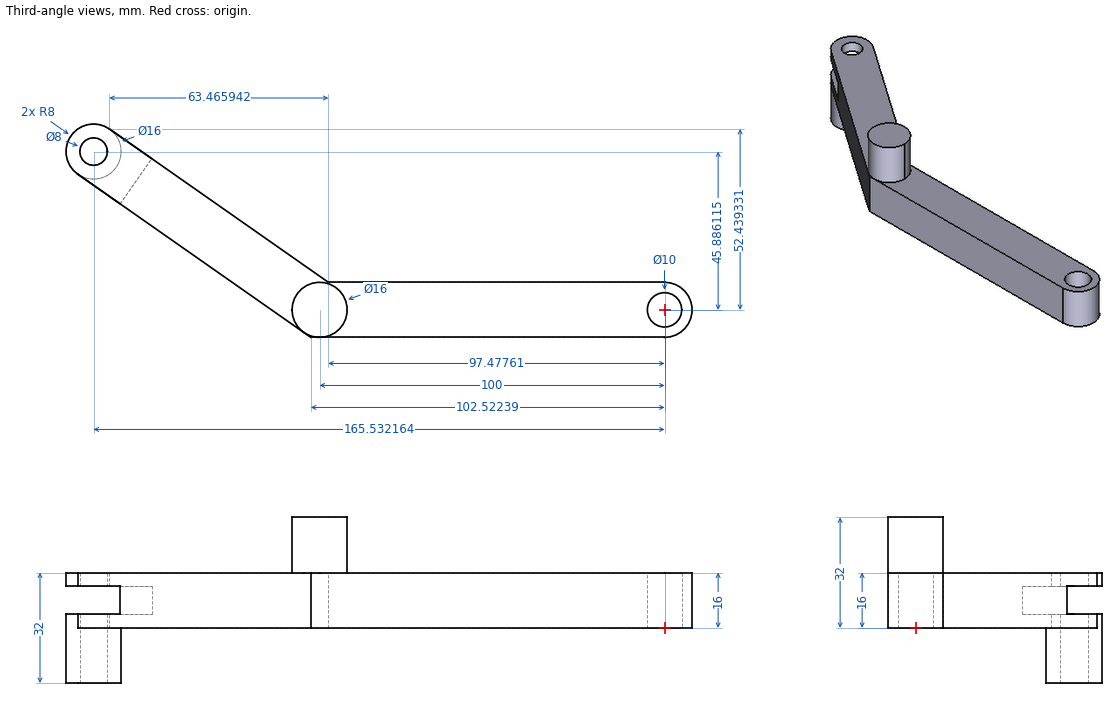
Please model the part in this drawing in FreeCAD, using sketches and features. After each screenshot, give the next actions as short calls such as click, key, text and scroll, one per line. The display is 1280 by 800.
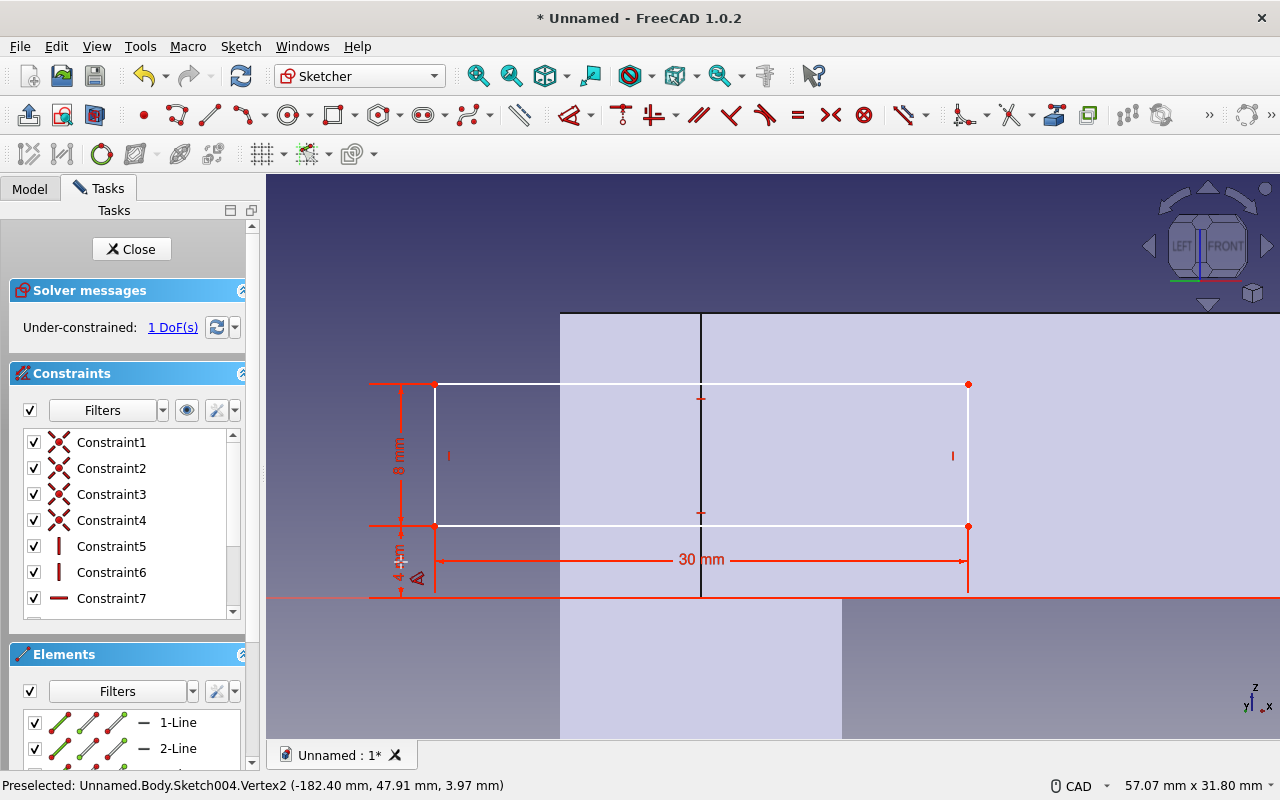
click(435, 384)
click(775, 632)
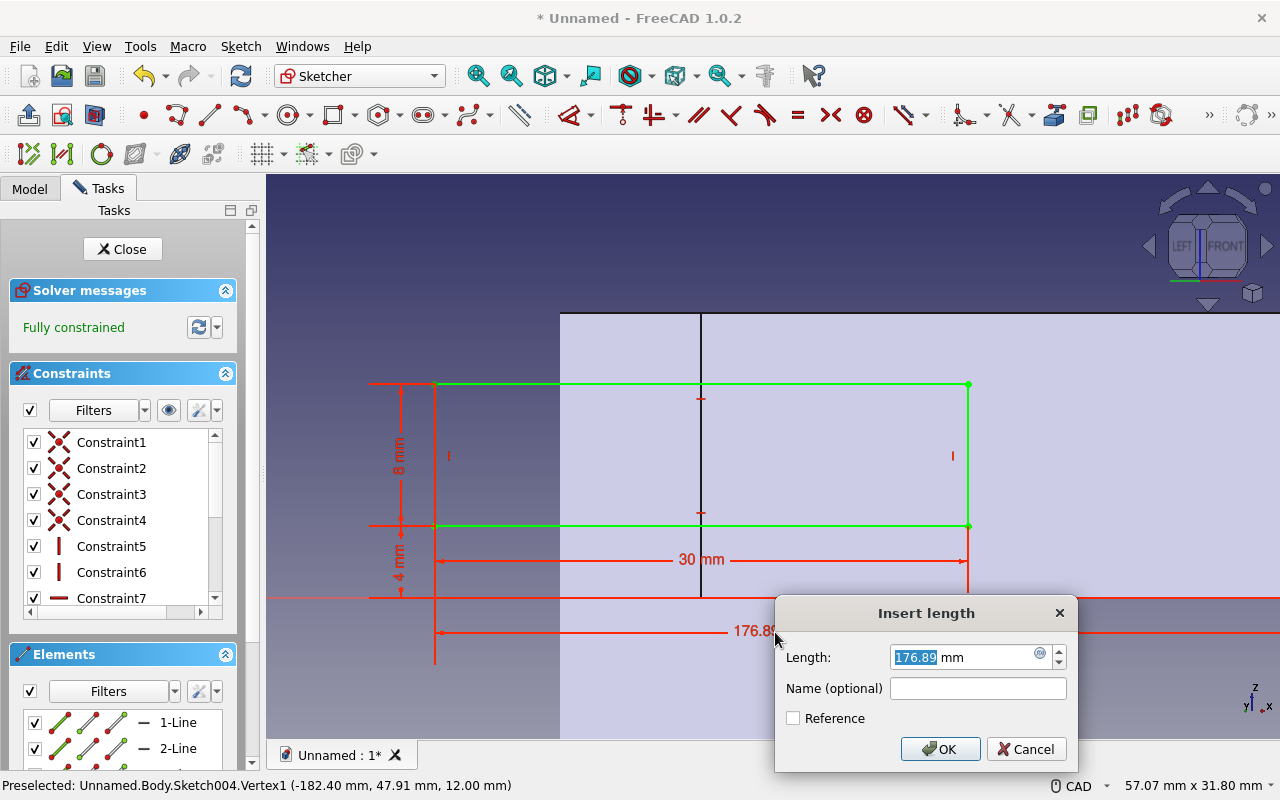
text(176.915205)
key(Return)
key(Escape)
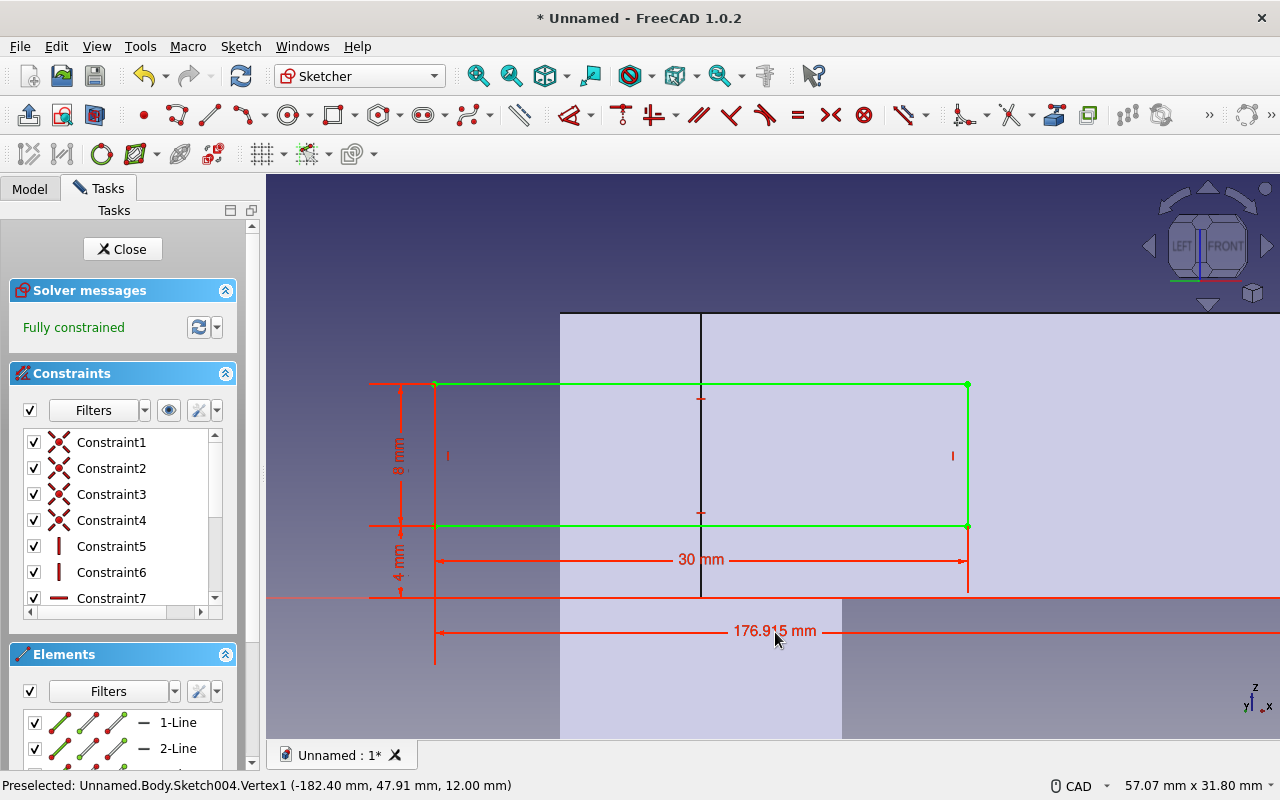
click(123, 249)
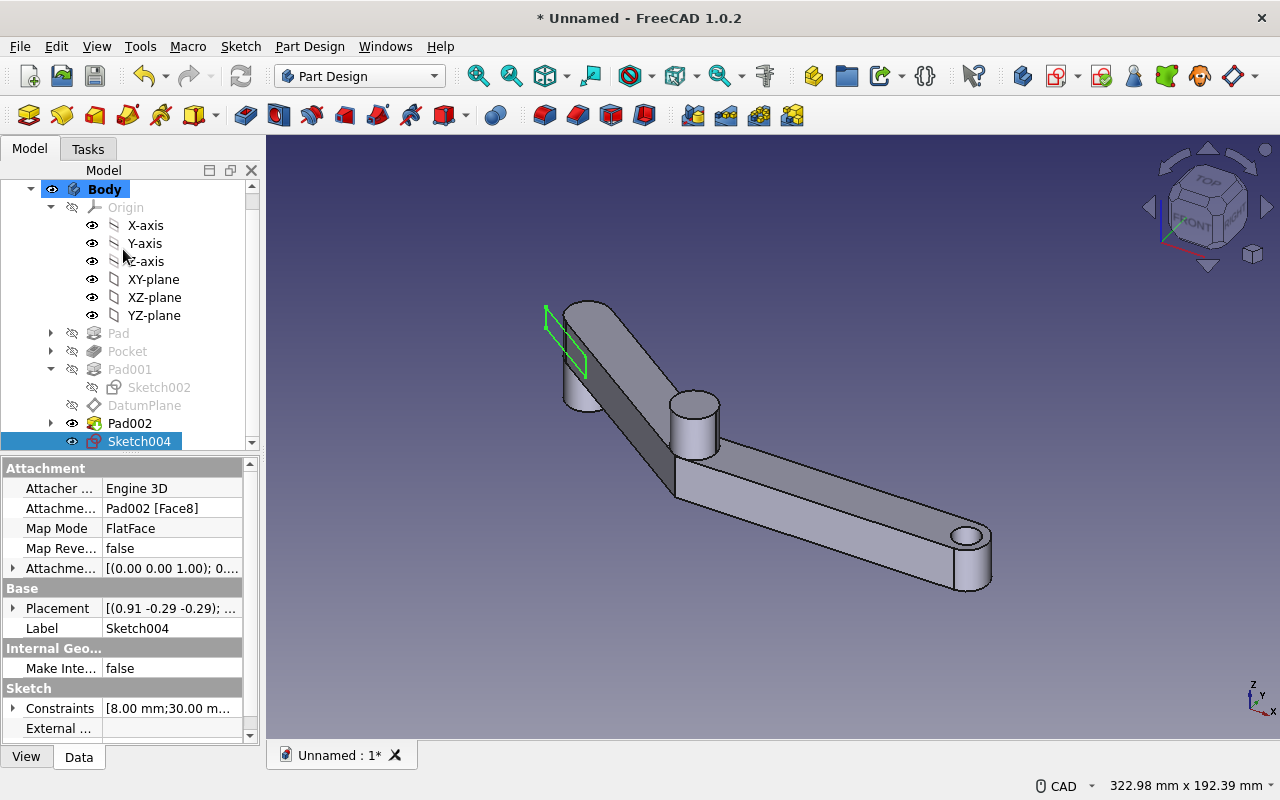
click(246, 116)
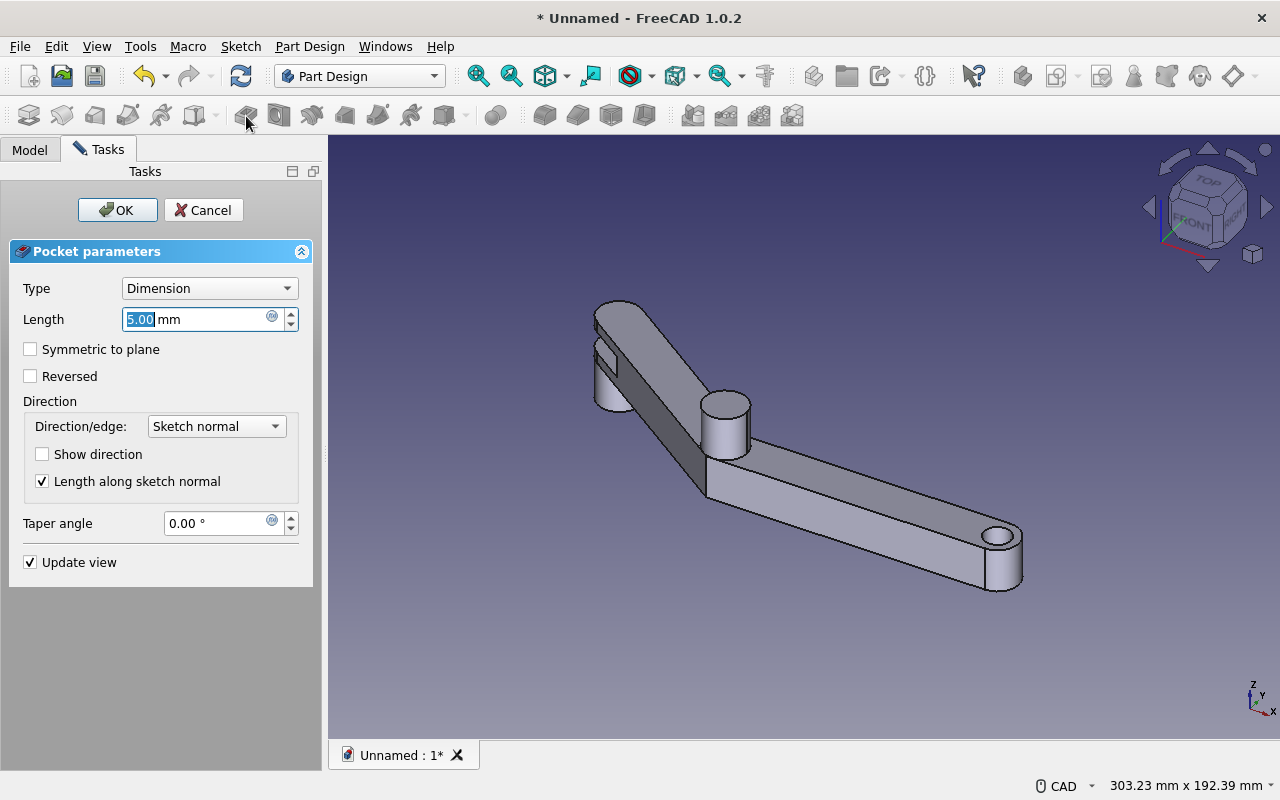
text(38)
key(Tab)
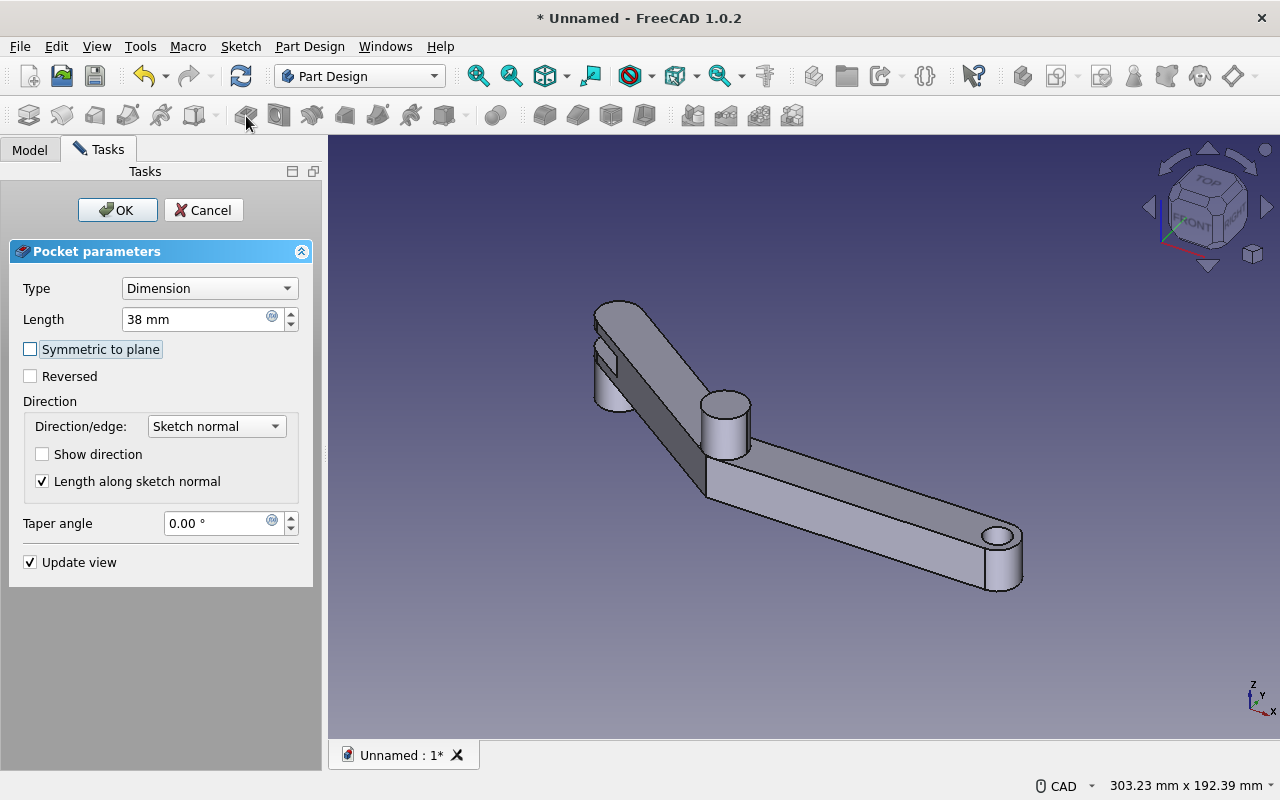
click(118, 210)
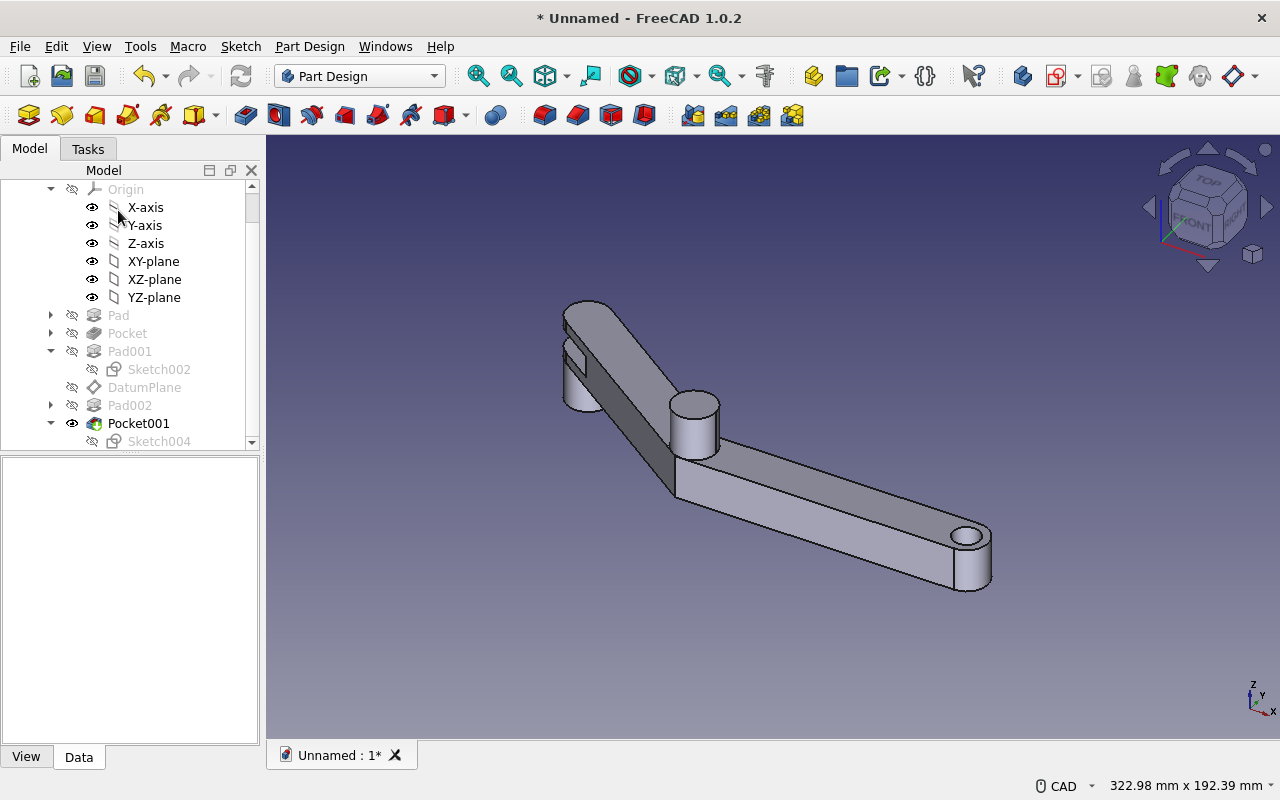
click(636, 378)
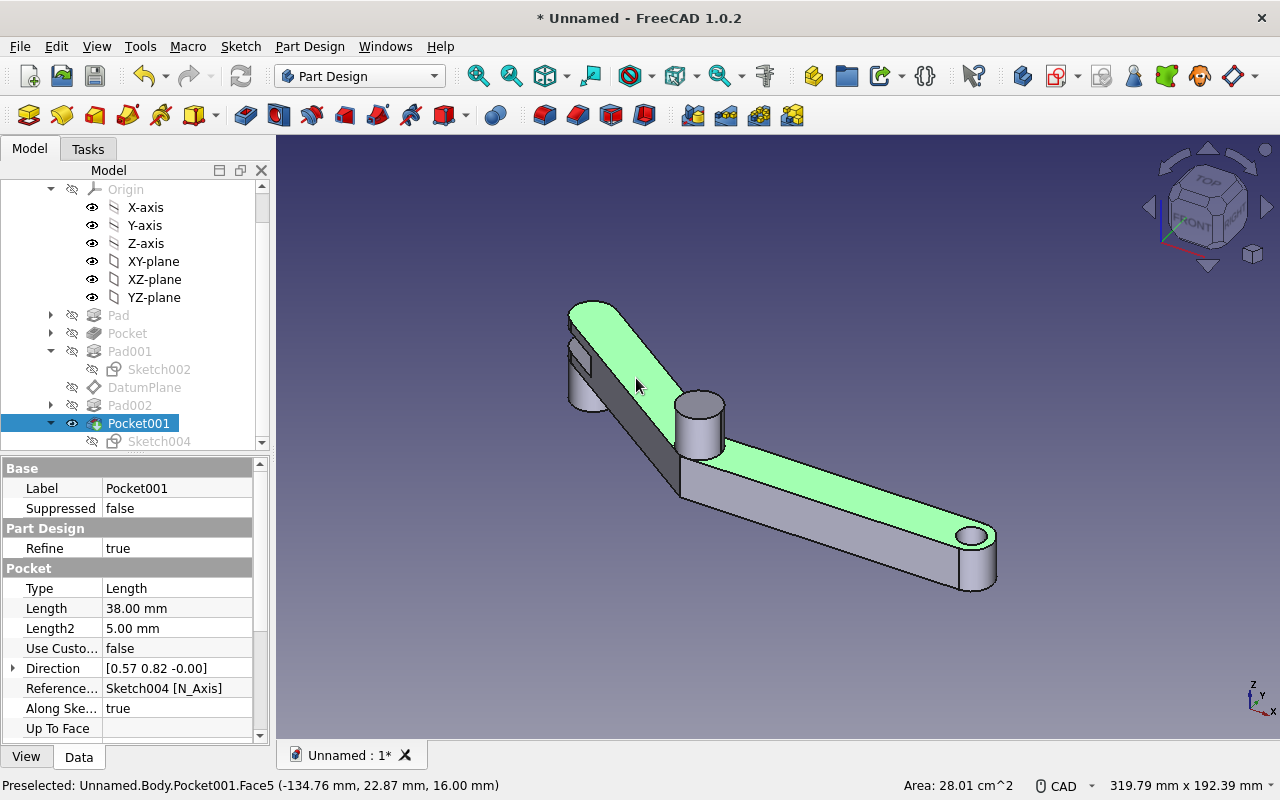
click(1056, 76)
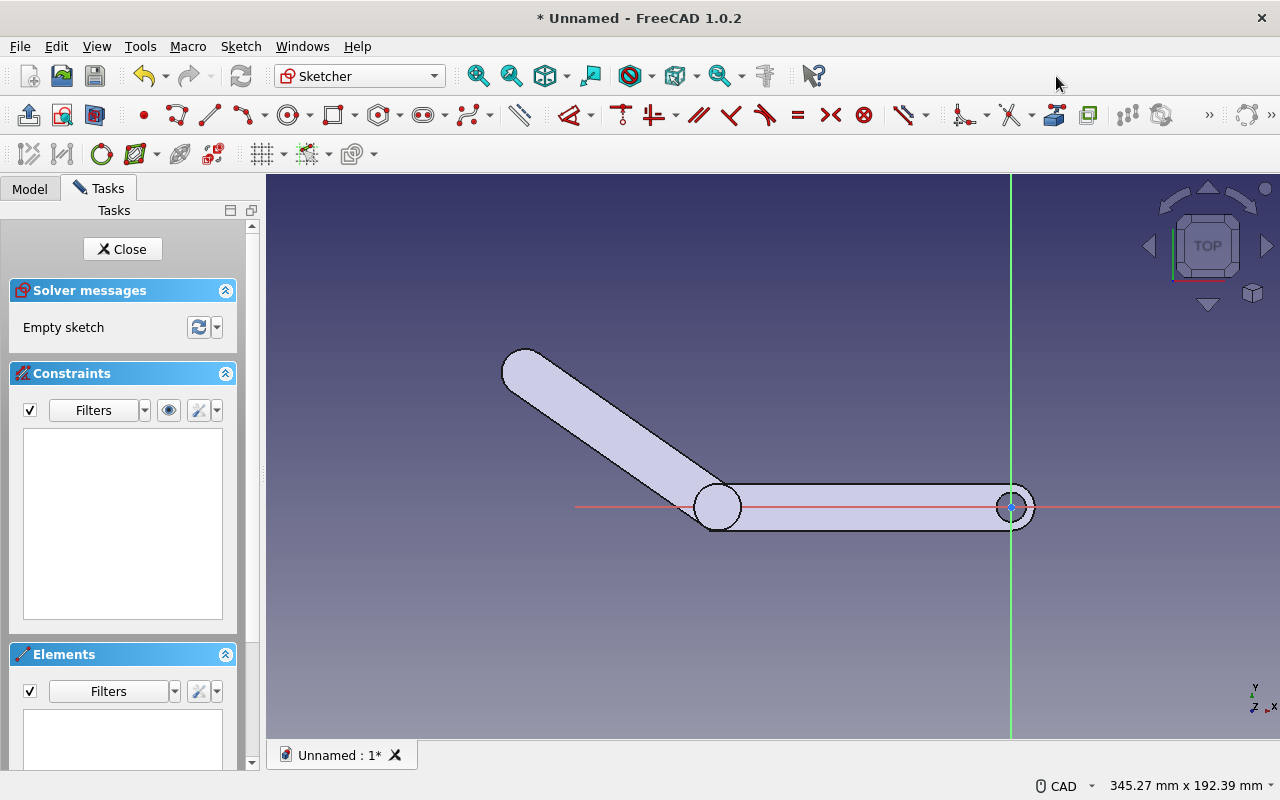
scroll(514, 367, up, 14)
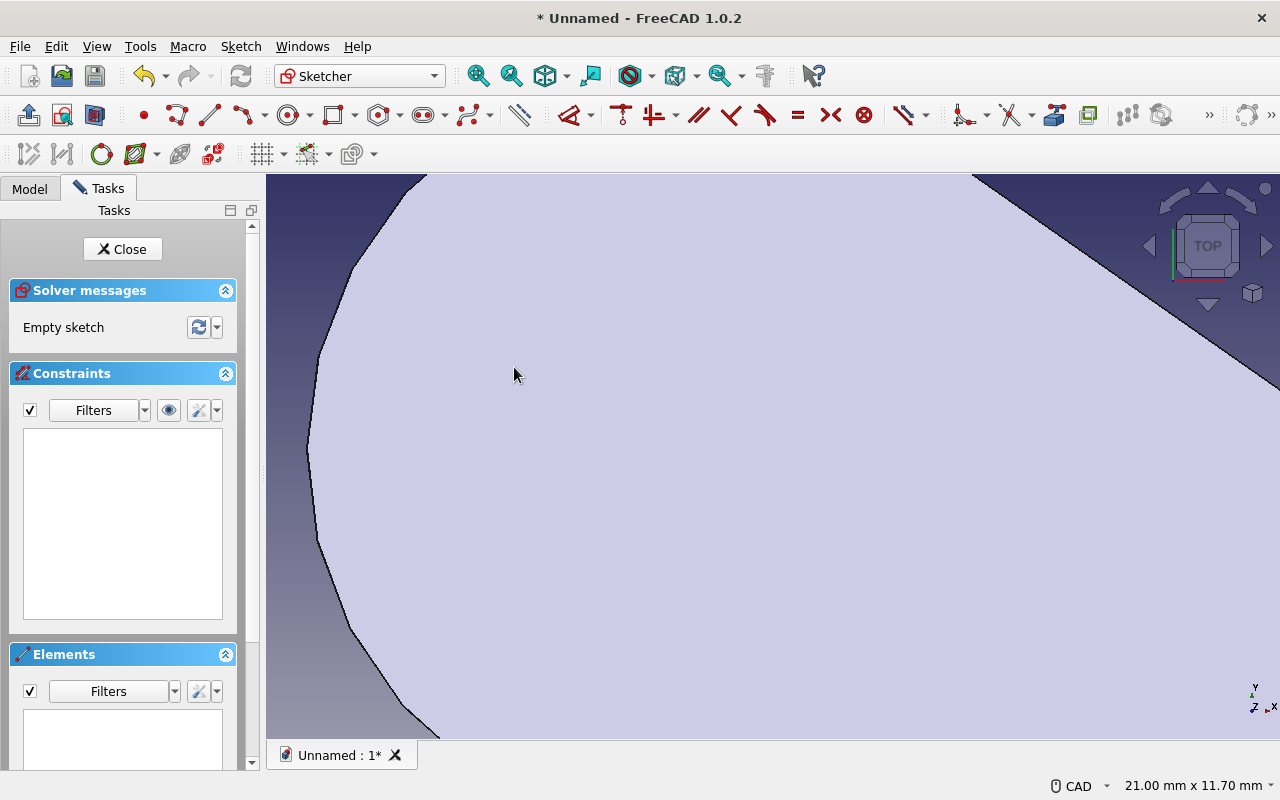
click(288, 116)